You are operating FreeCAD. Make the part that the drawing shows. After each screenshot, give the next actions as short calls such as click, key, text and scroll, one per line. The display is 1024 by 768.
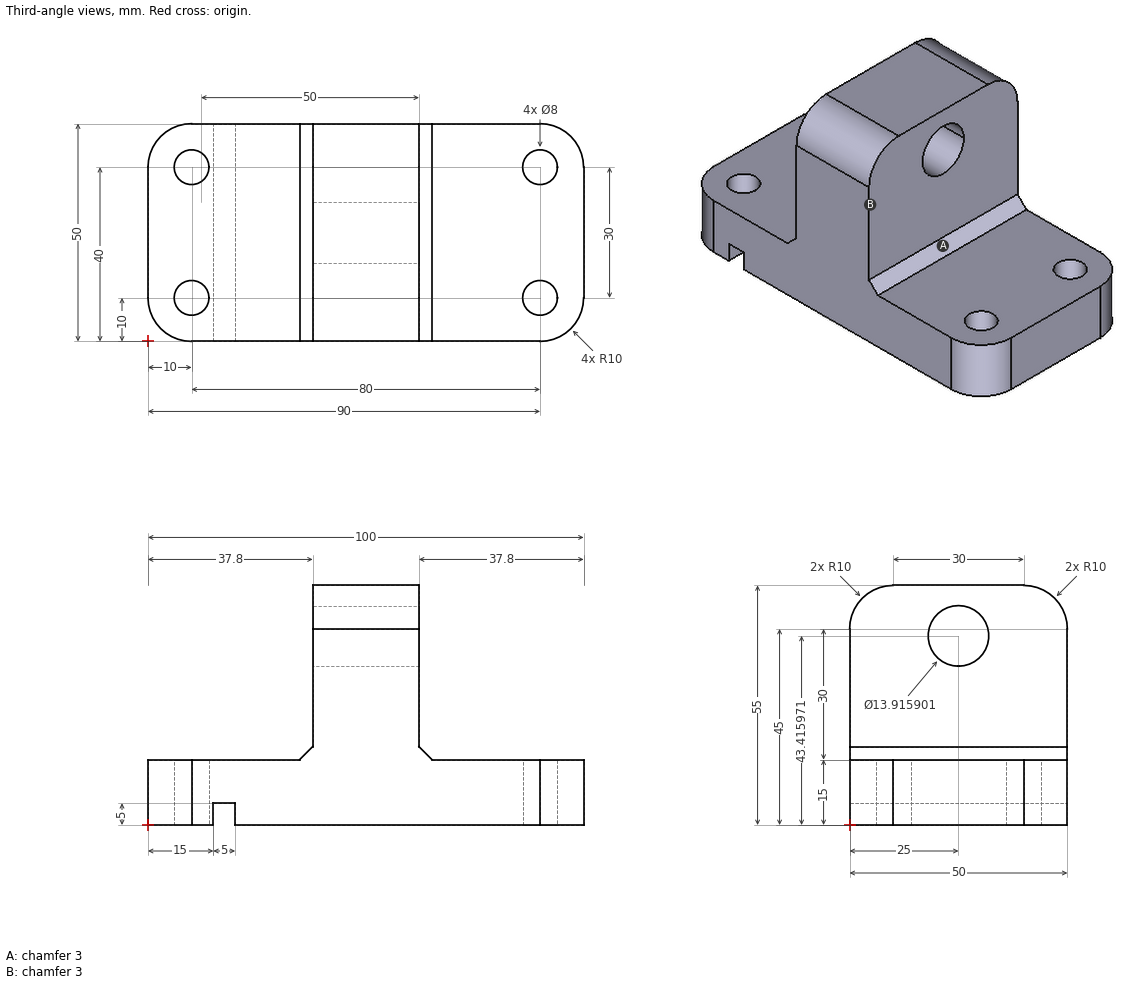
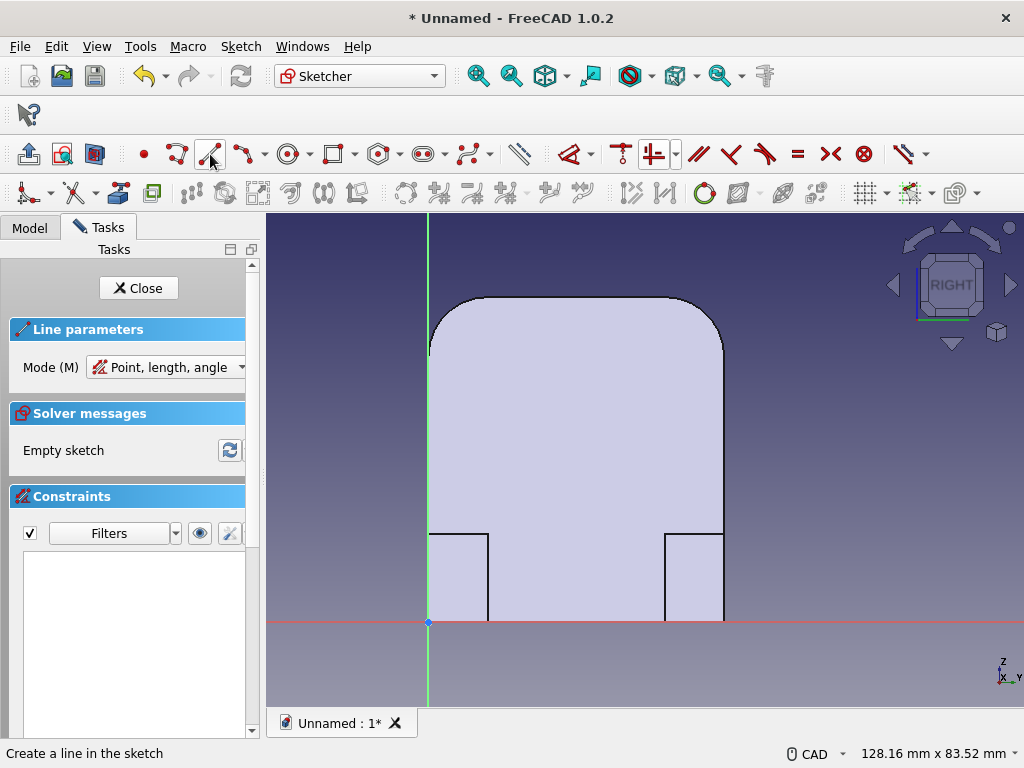
click(665, 297)
click(488, 297)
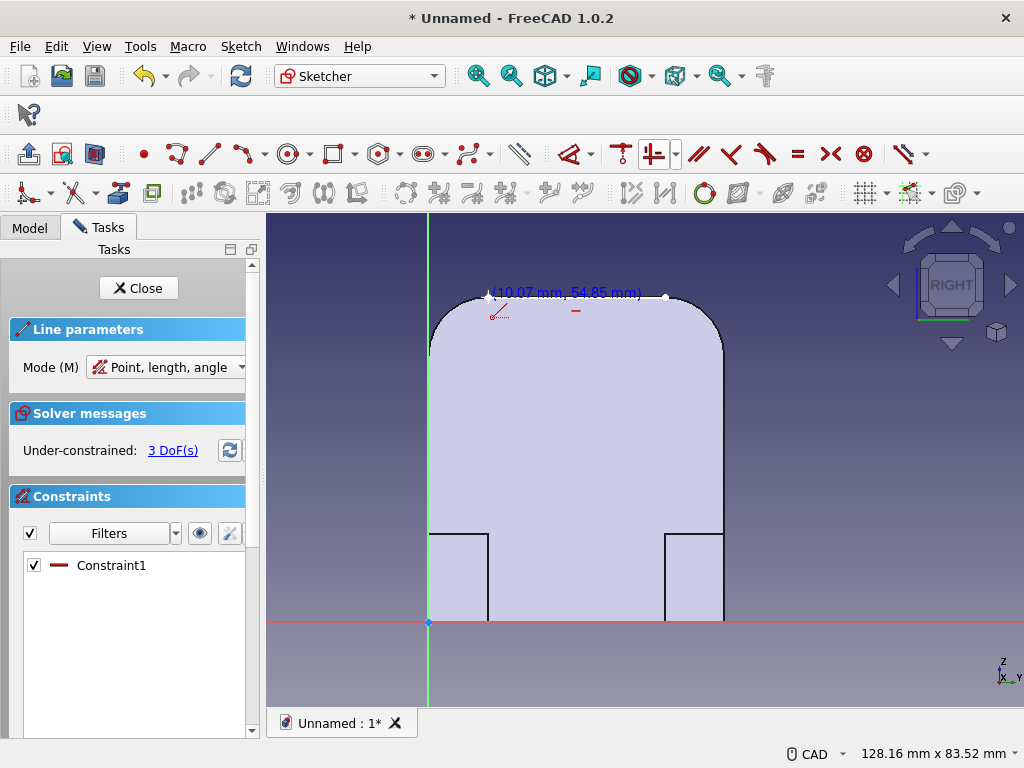
click(177, 154)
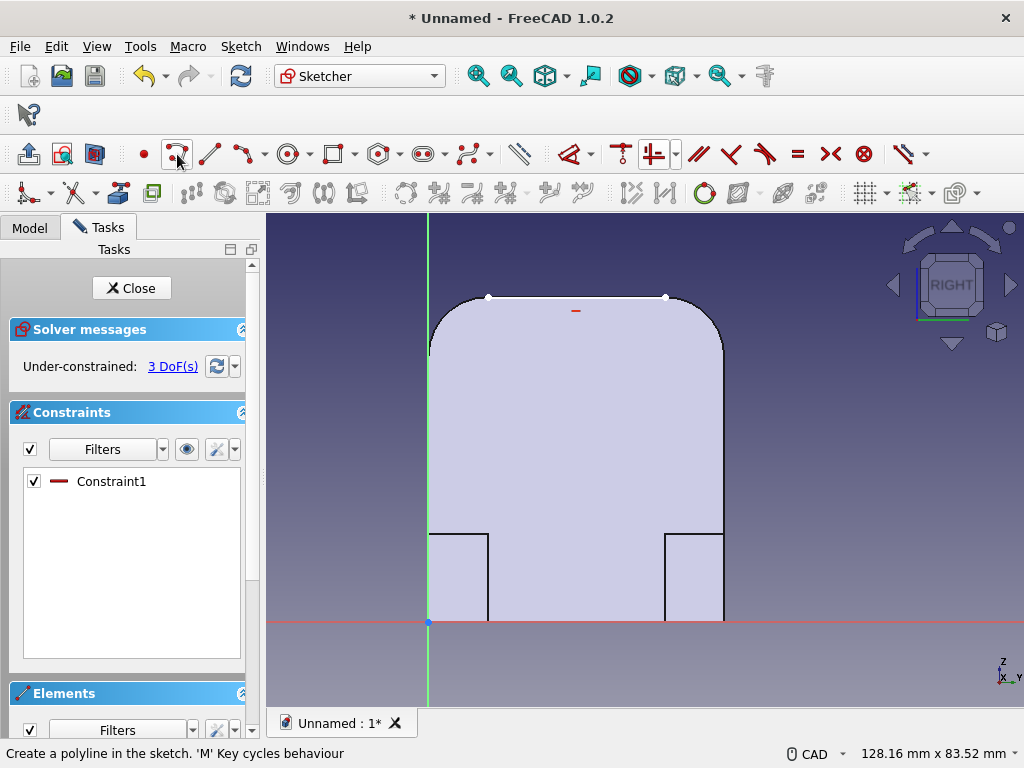
click(428, 356)
click(437, 534)
click(724, 534)
click(724, 356)
right_click(724, 356)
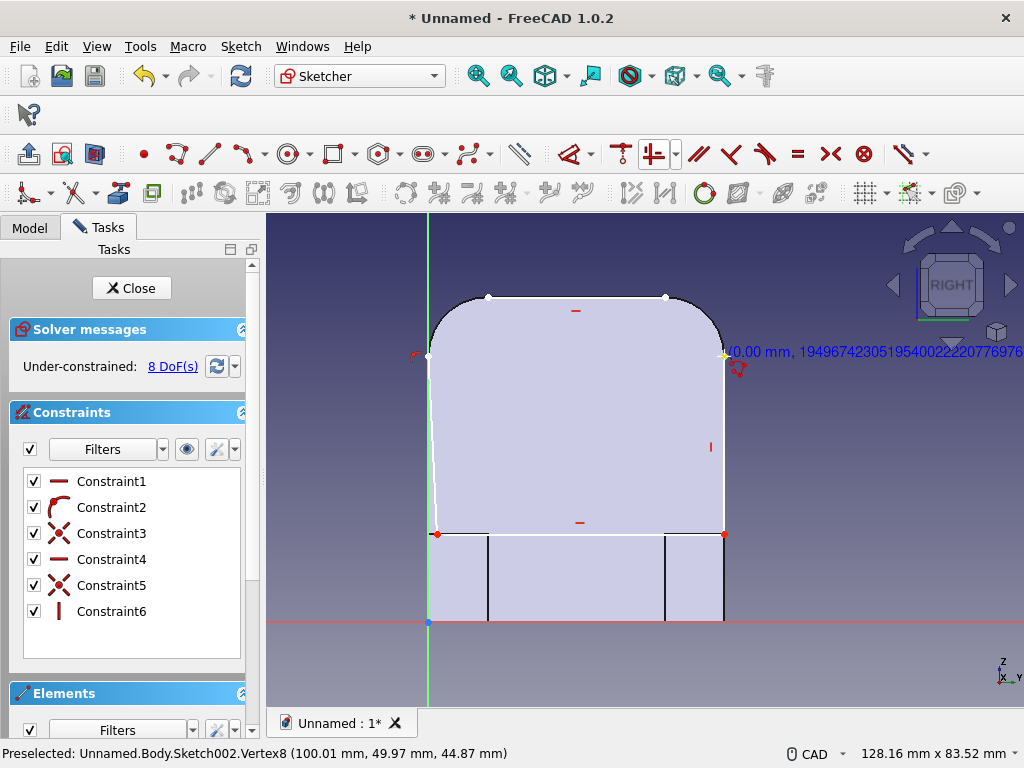
click(242, 154)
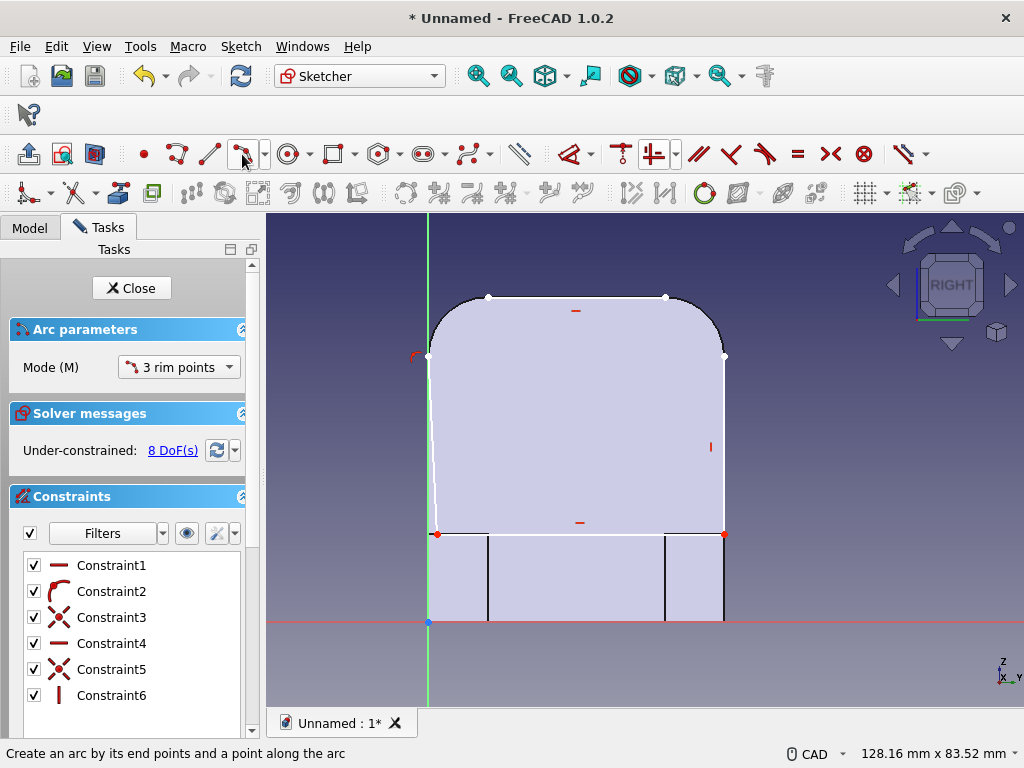
click(488, 298)
click(428, 357)
click(446, 314)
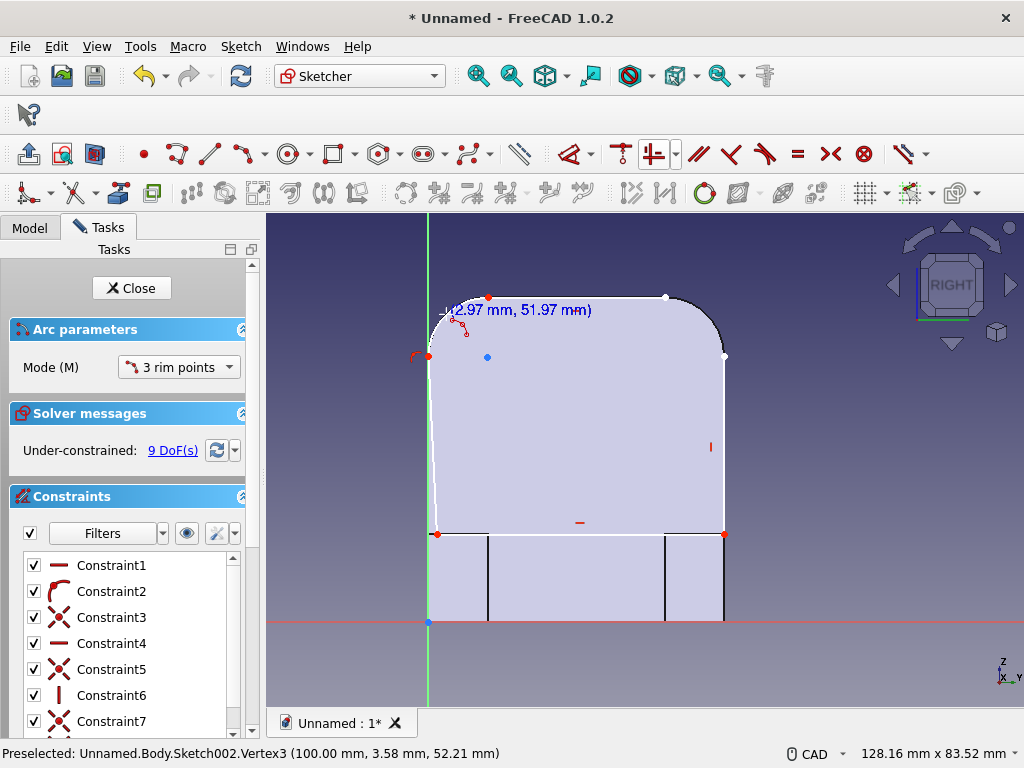
click(724, 357)
click(665, 298)
click(707, 314)
key(Escape)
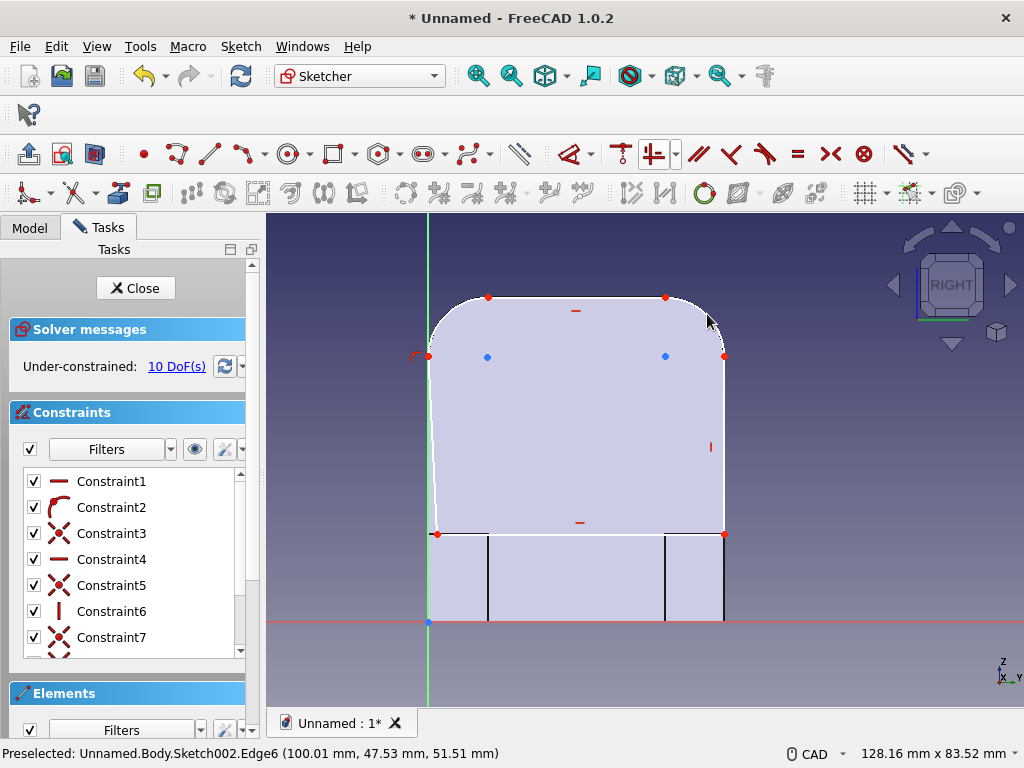
click(612, 298)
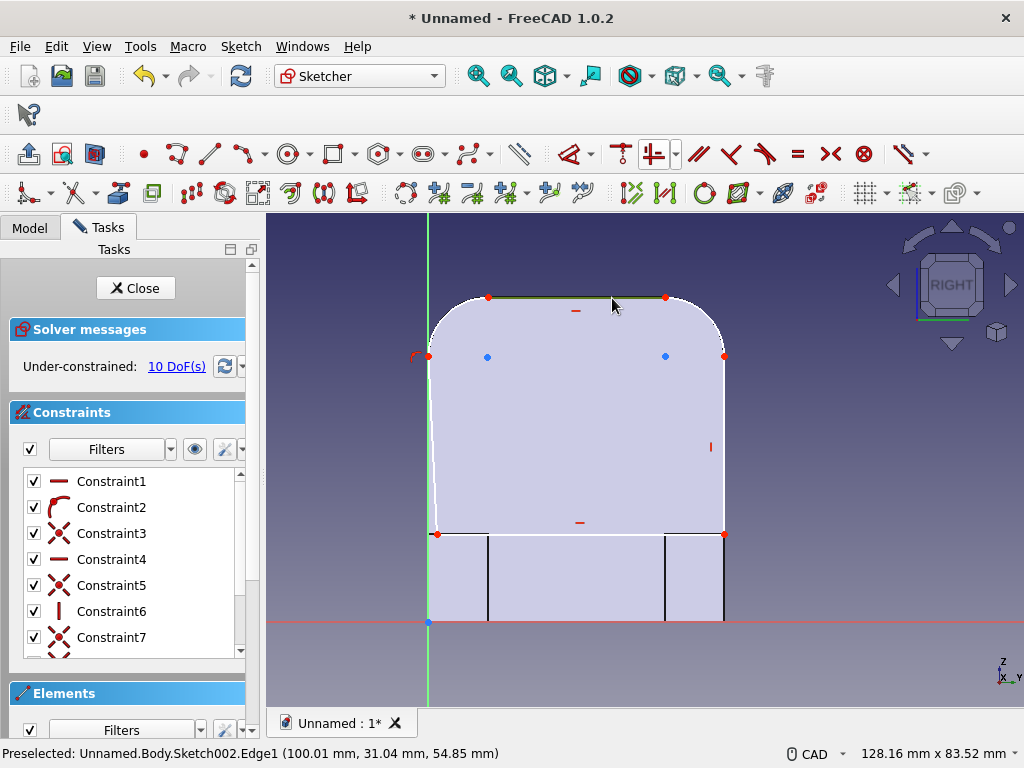
click(461, 304)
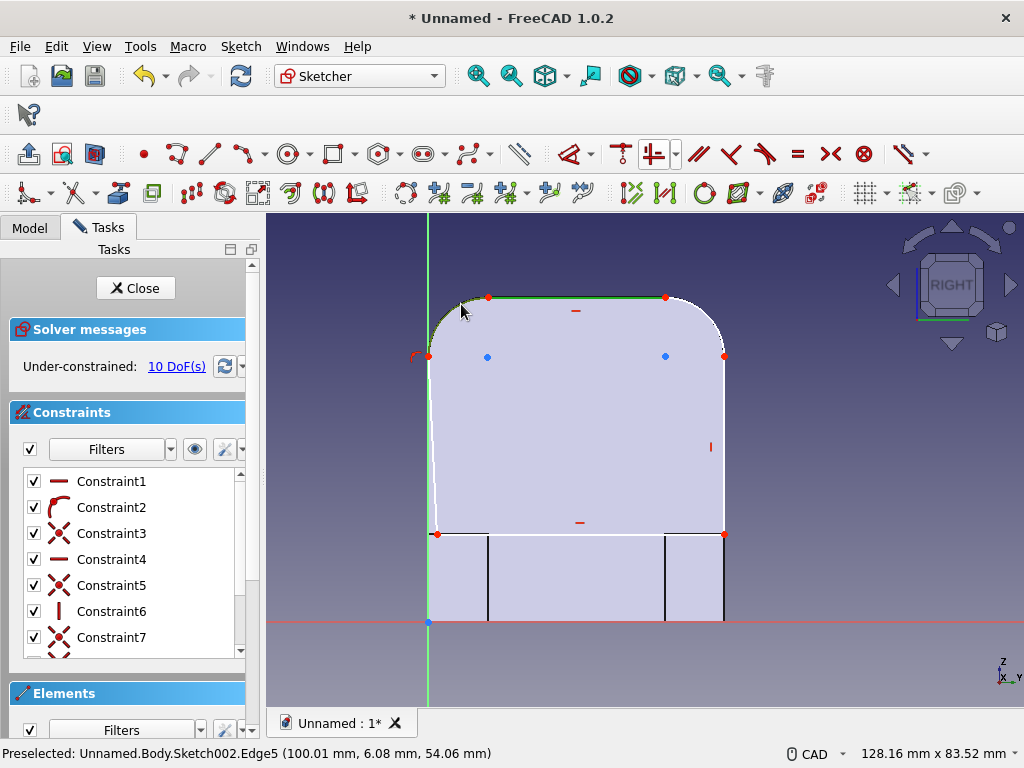
click(765, 154)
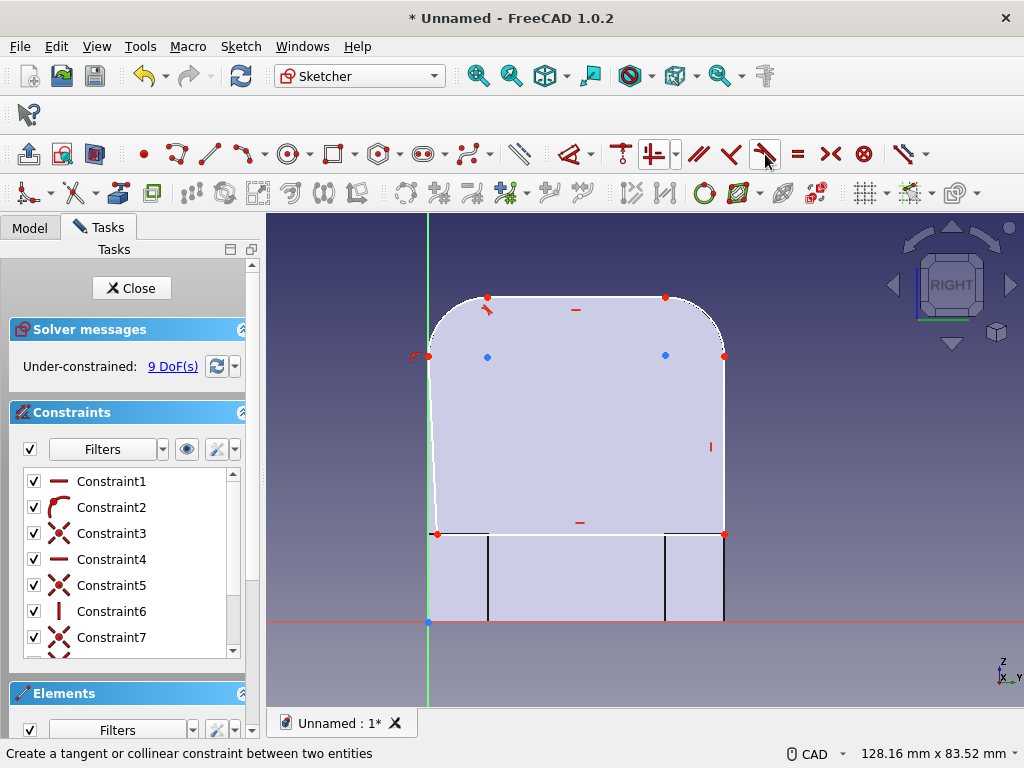
click(612, 297)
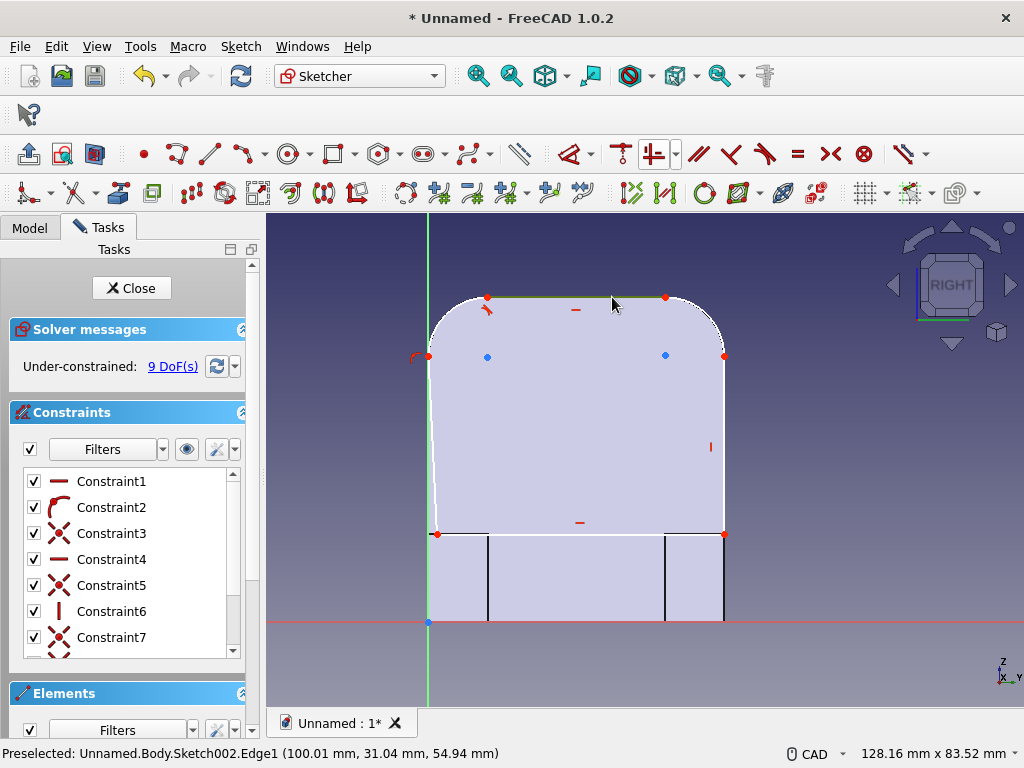
click(718, 330)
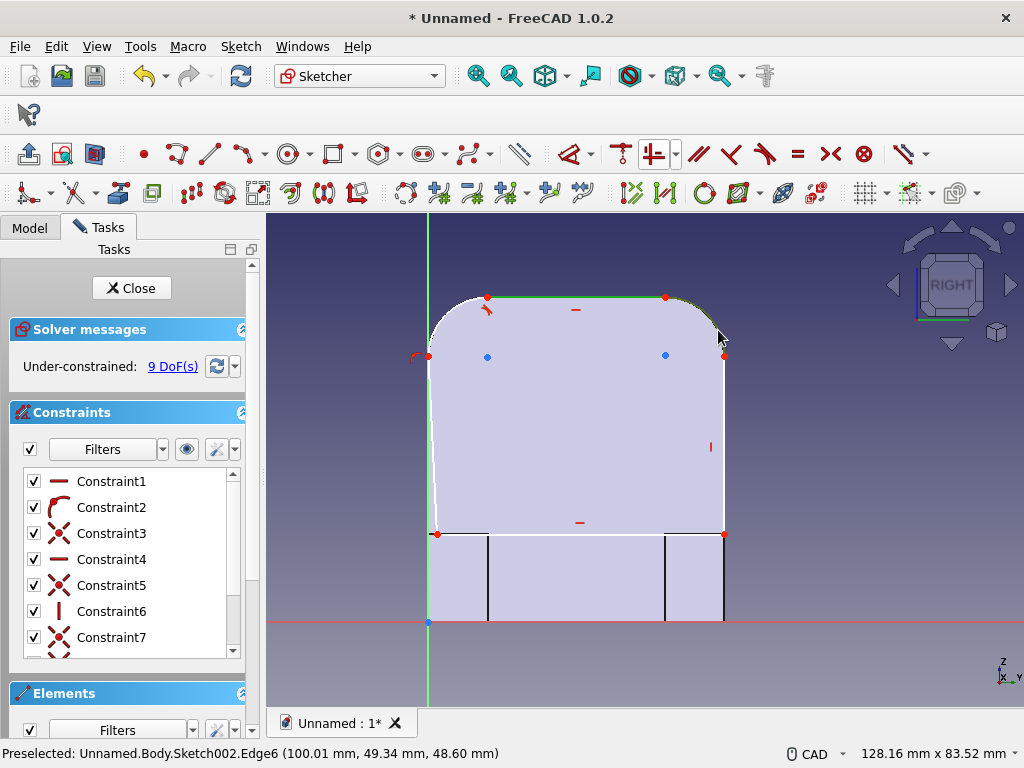
click(765, 154)